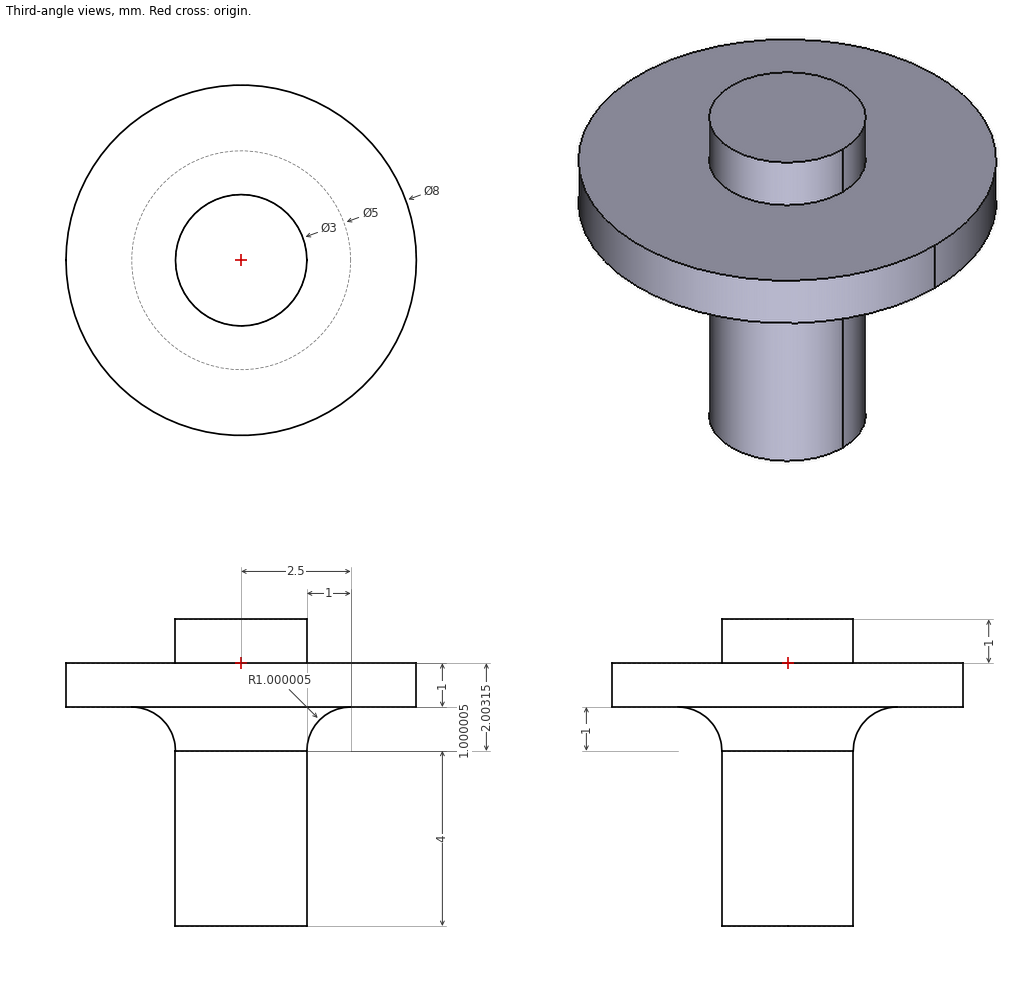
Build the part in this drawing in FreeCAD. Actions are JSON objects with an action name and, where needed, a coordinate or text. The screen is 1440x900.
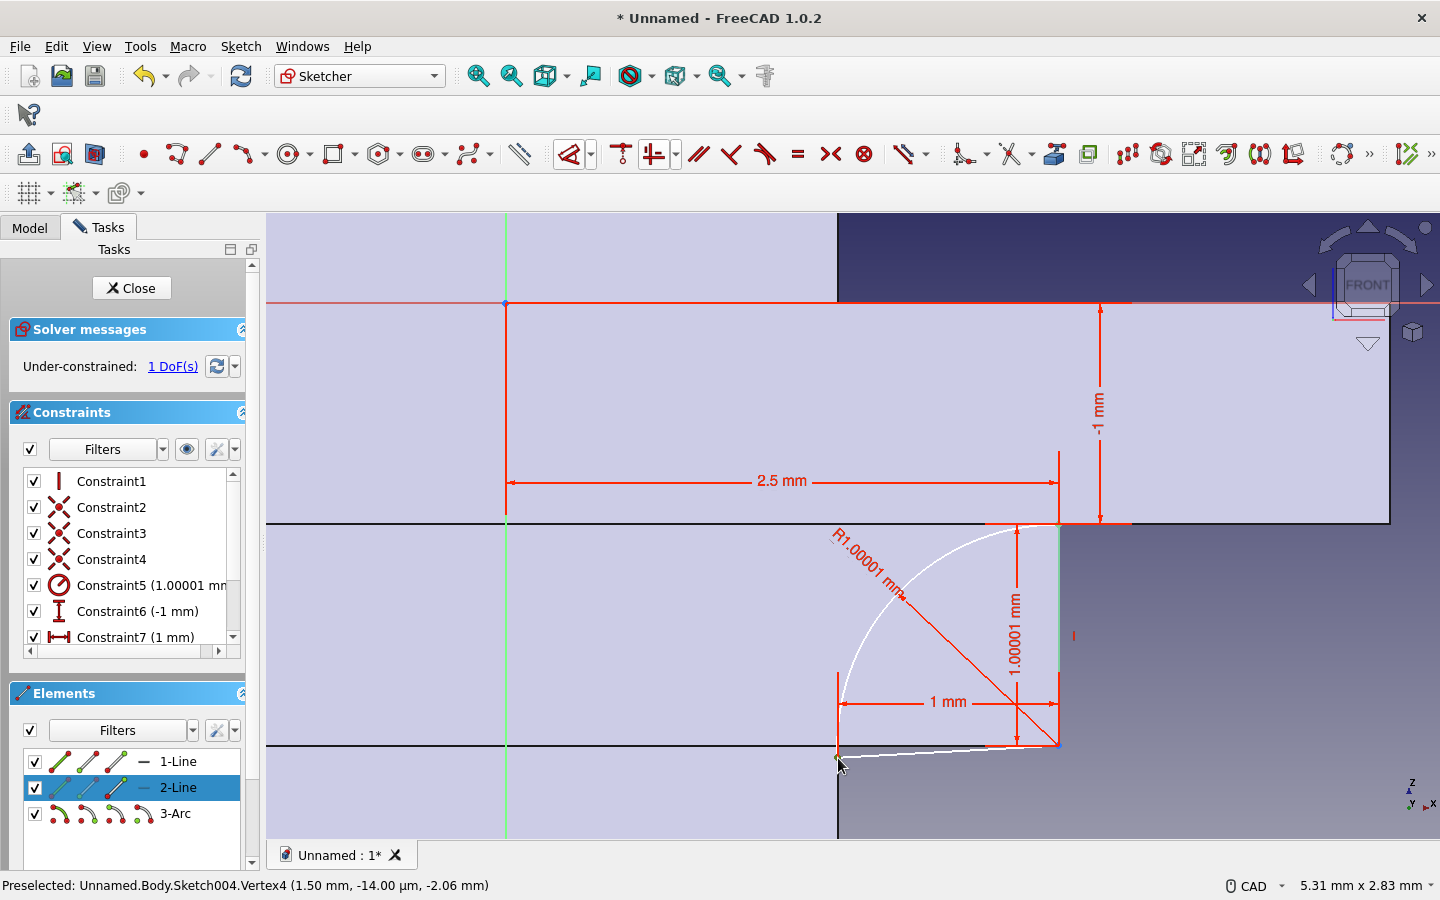
{"action": "key", "text": "i"}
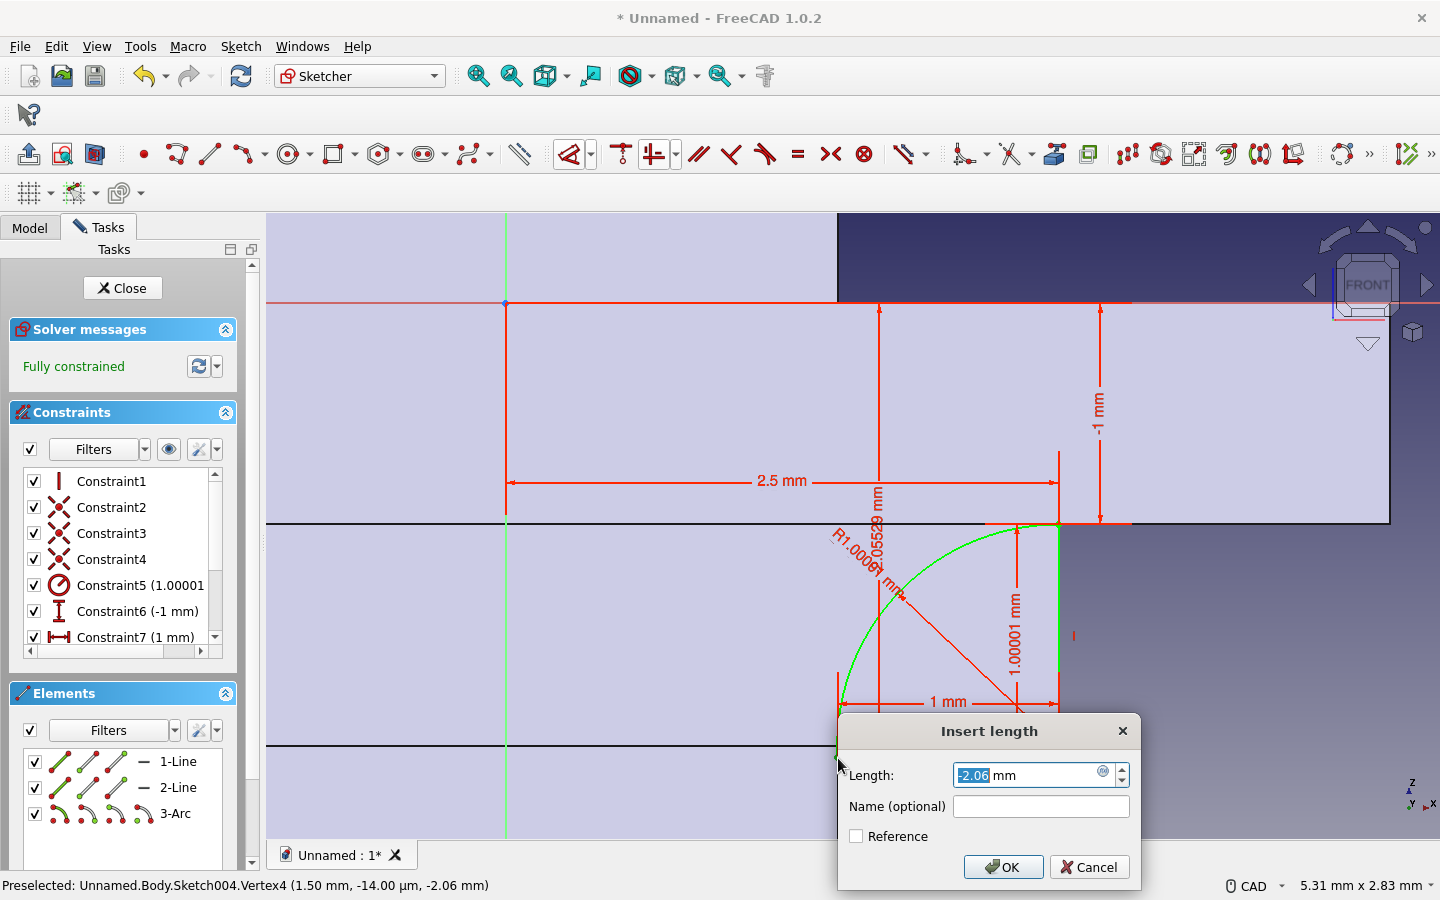
{"action": "type", "text": "-2.00315"}
{"action": "key", "text": "Return"}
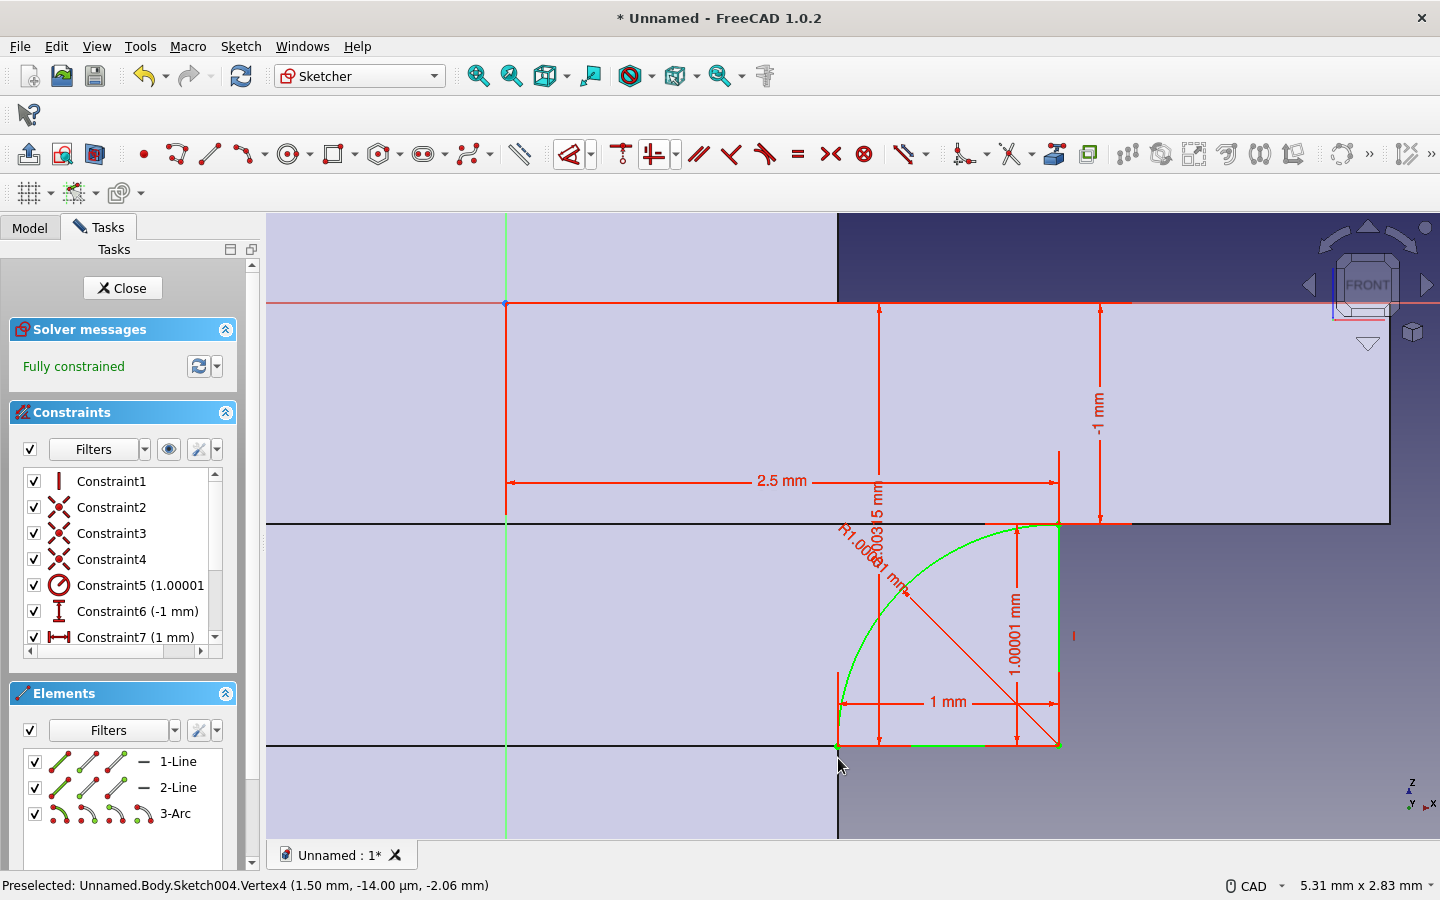
{"action": "left_click", "coordinate": [123, 288]}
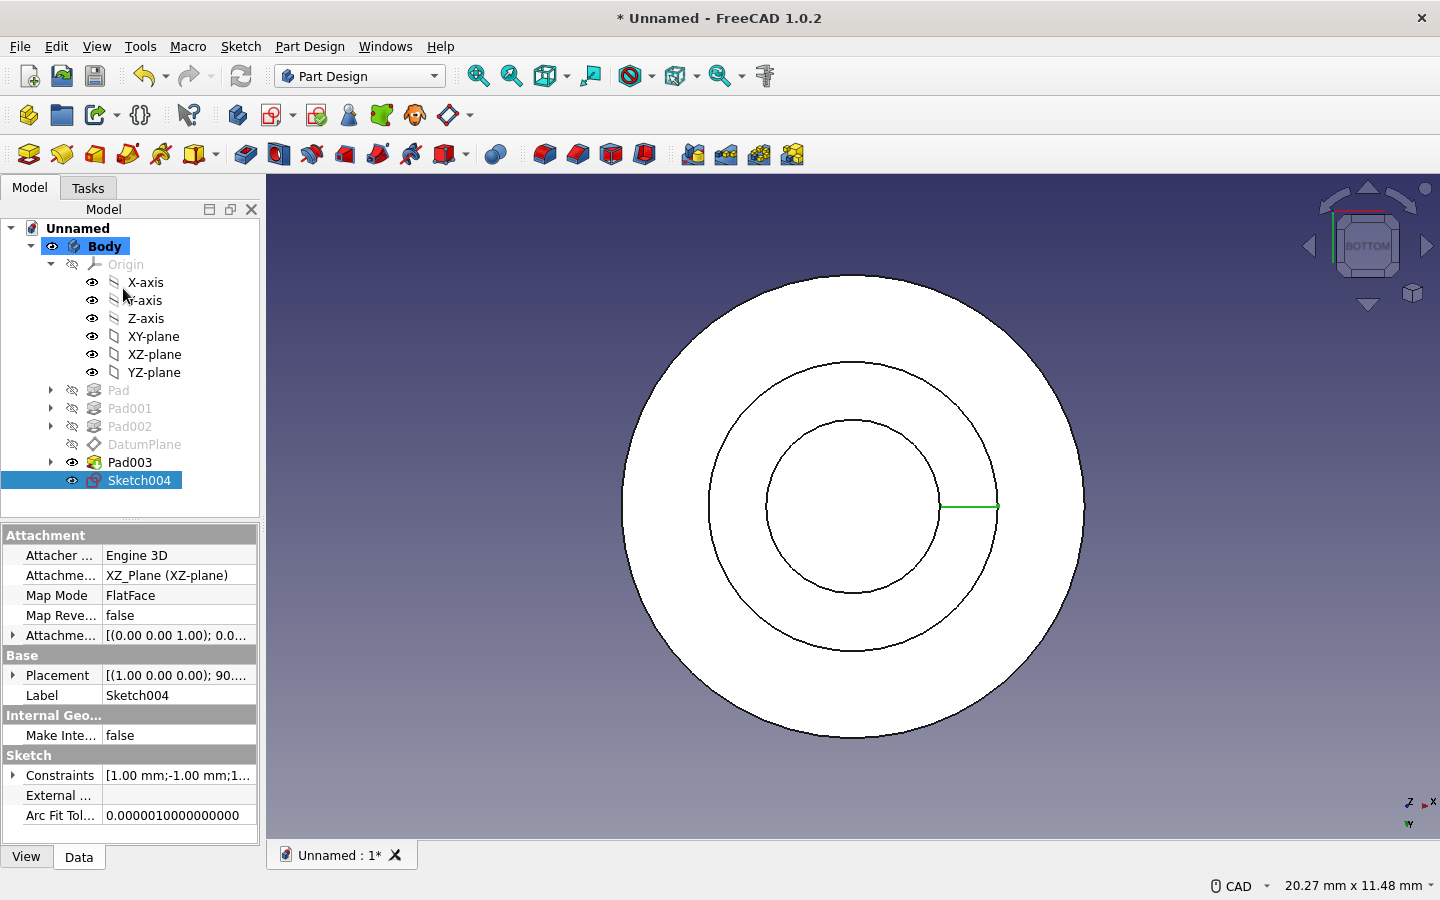
{"action": "left_click", "coordinate": [312, 154]}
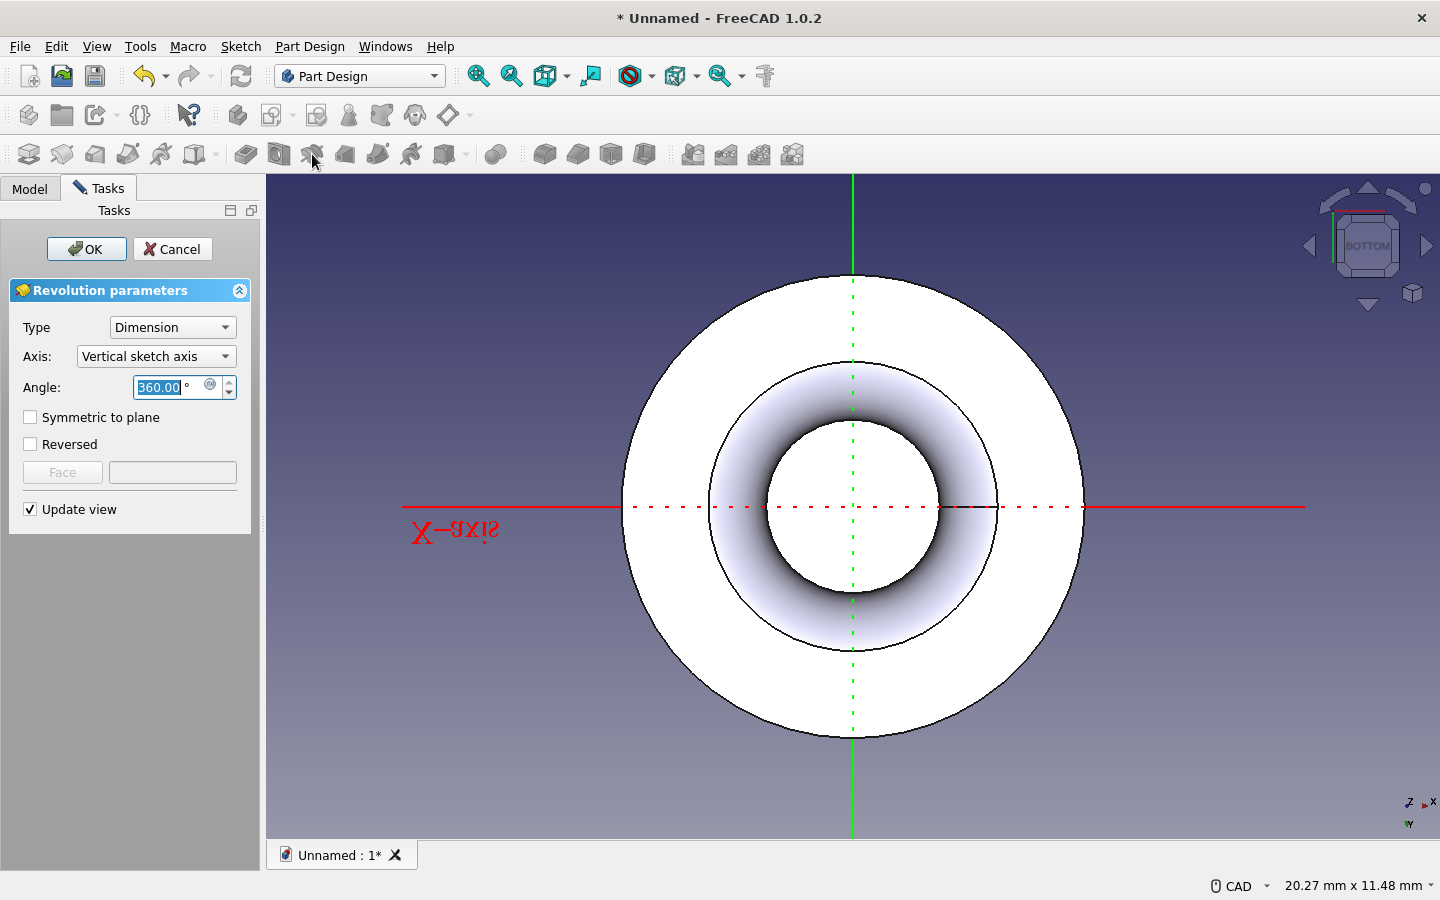
{"action": "left_click", "coordinate": [87, 249]}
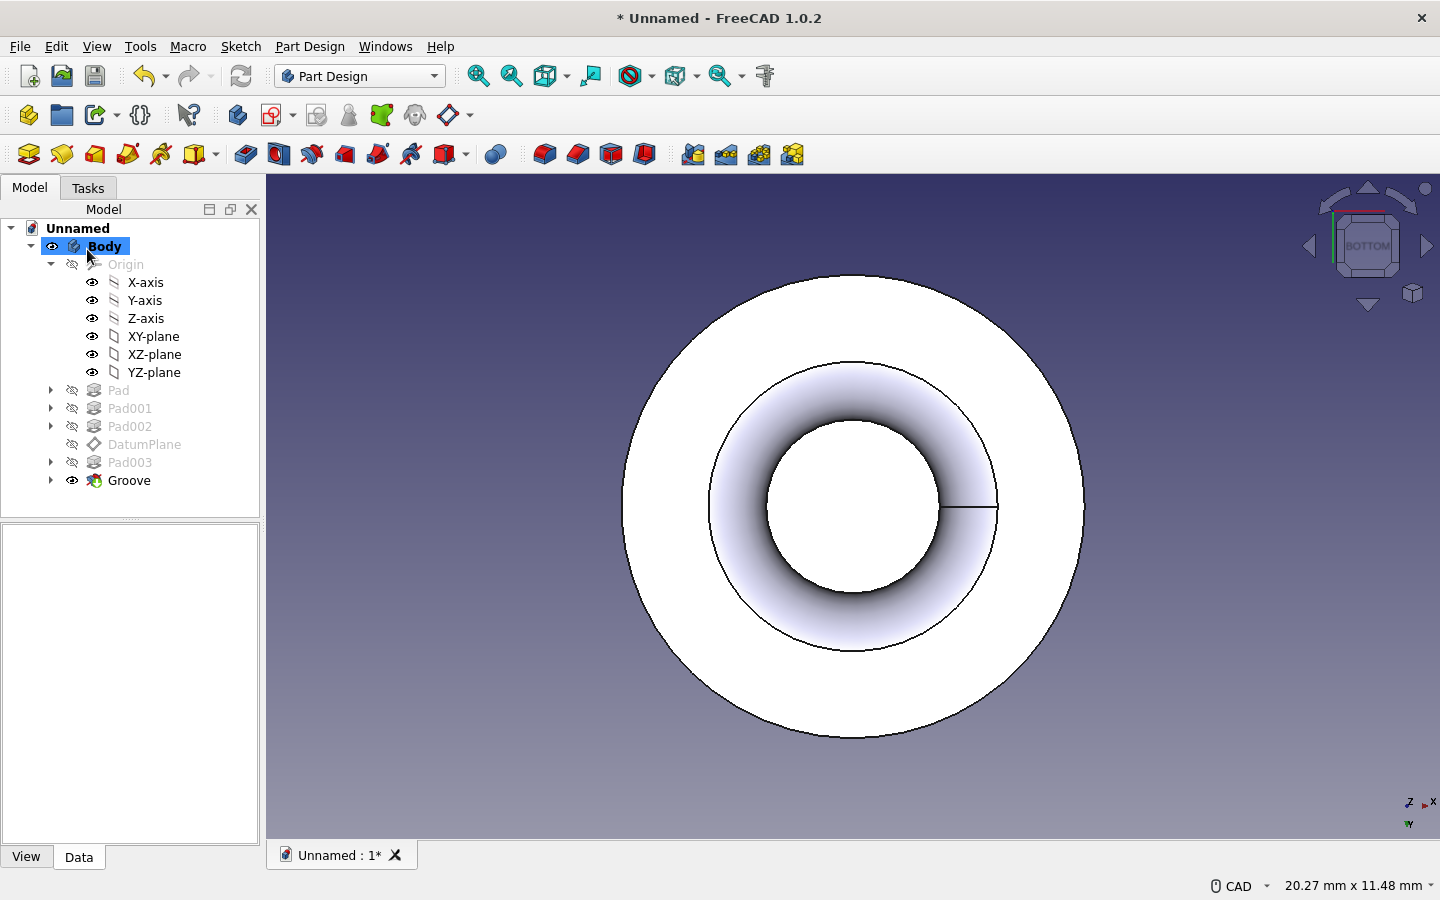
{"action": "key", "text": "0"}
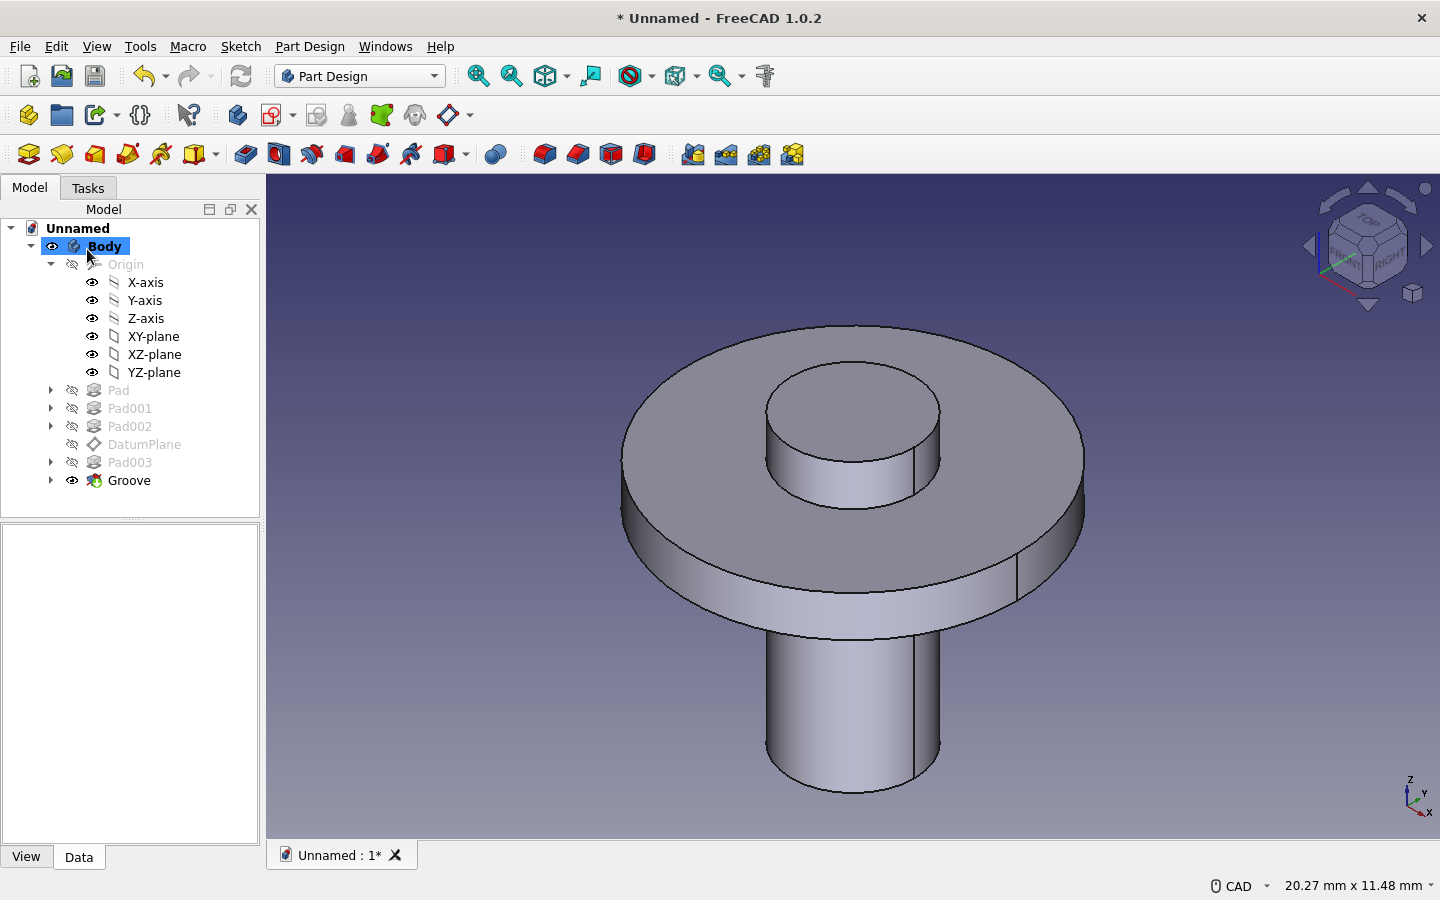
{"action": "left_click", "coordinate": [479, 76]}